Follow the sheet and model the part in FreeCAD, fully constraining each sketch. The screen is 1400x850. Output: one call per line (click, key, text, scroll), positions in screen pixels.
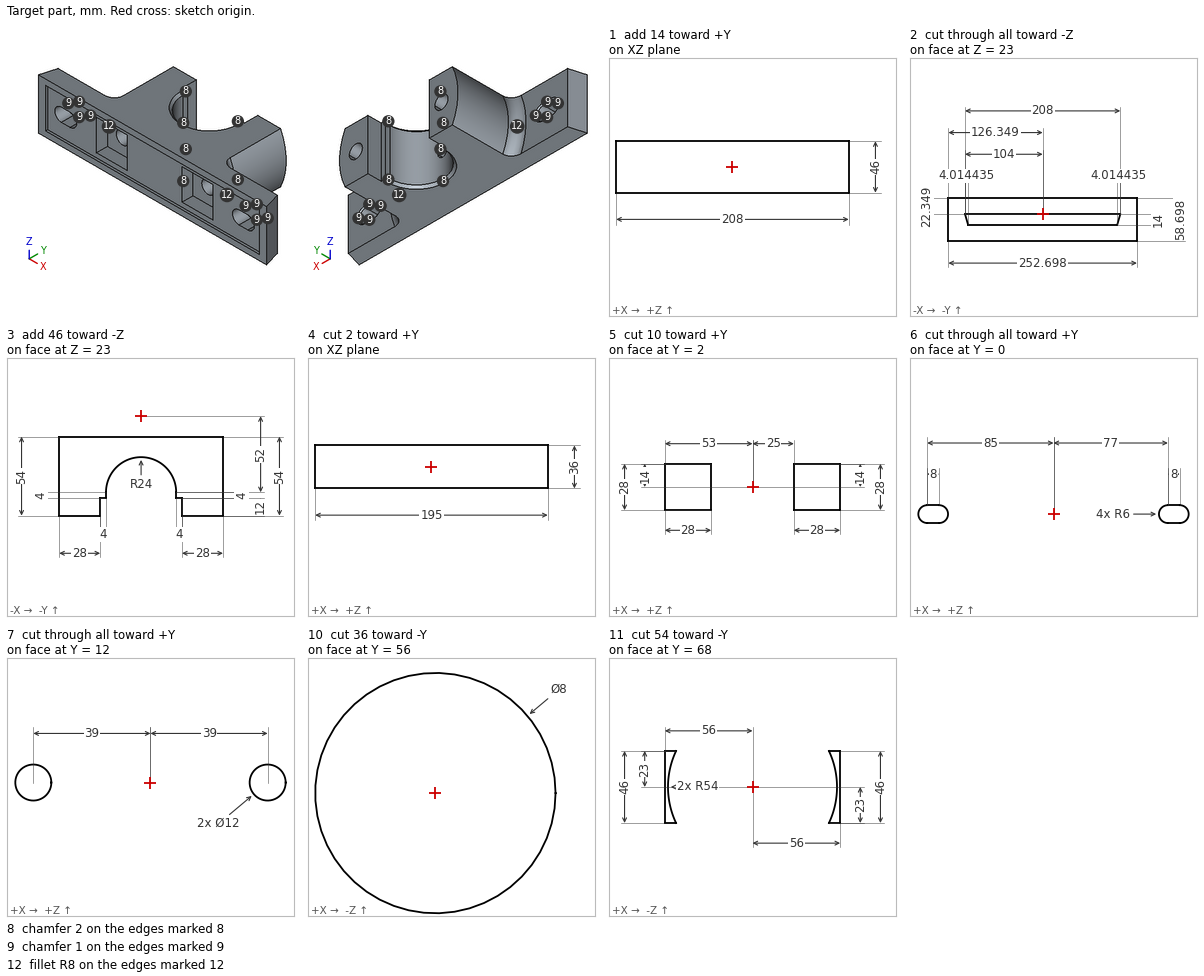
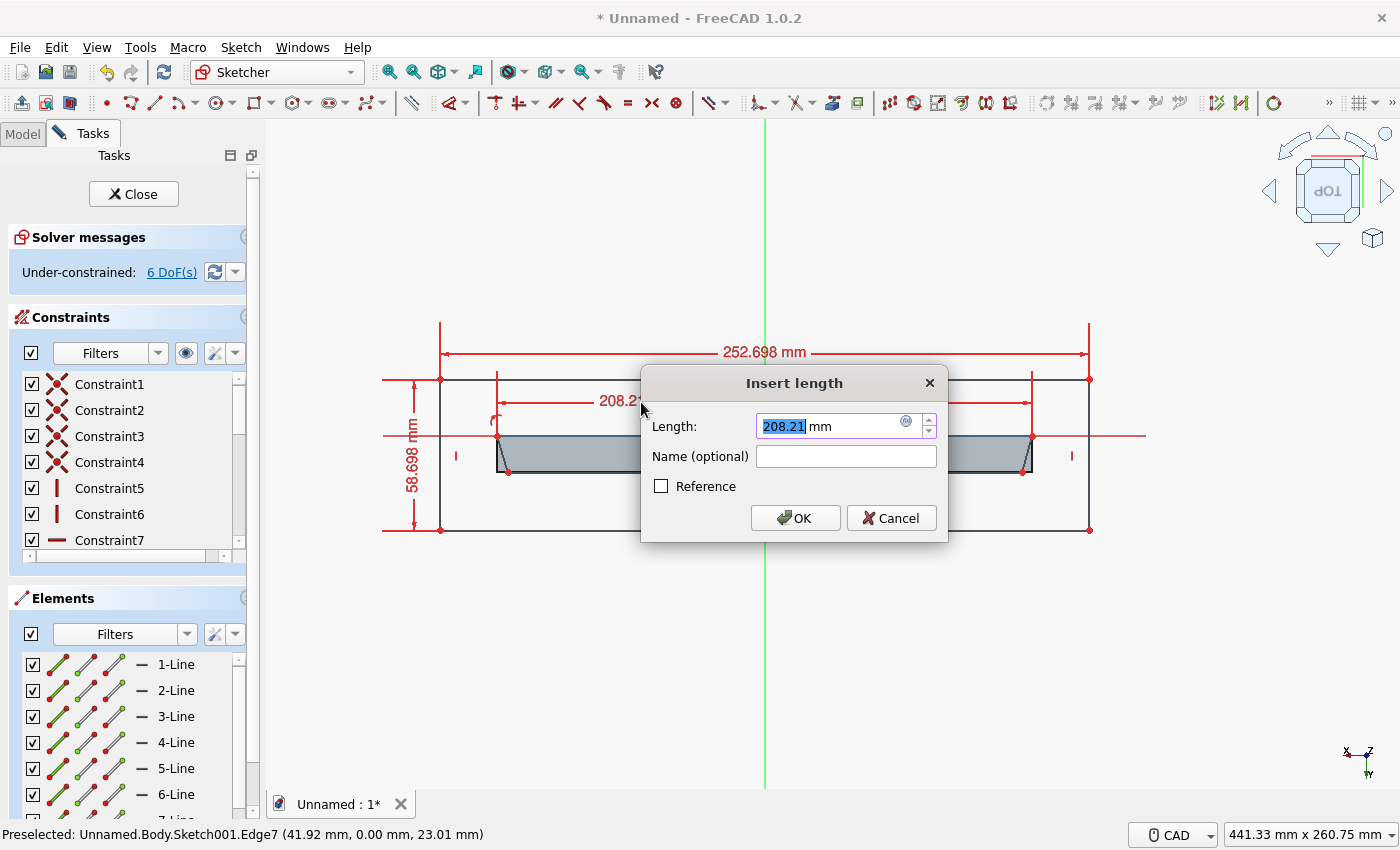
text(208)
key(Return)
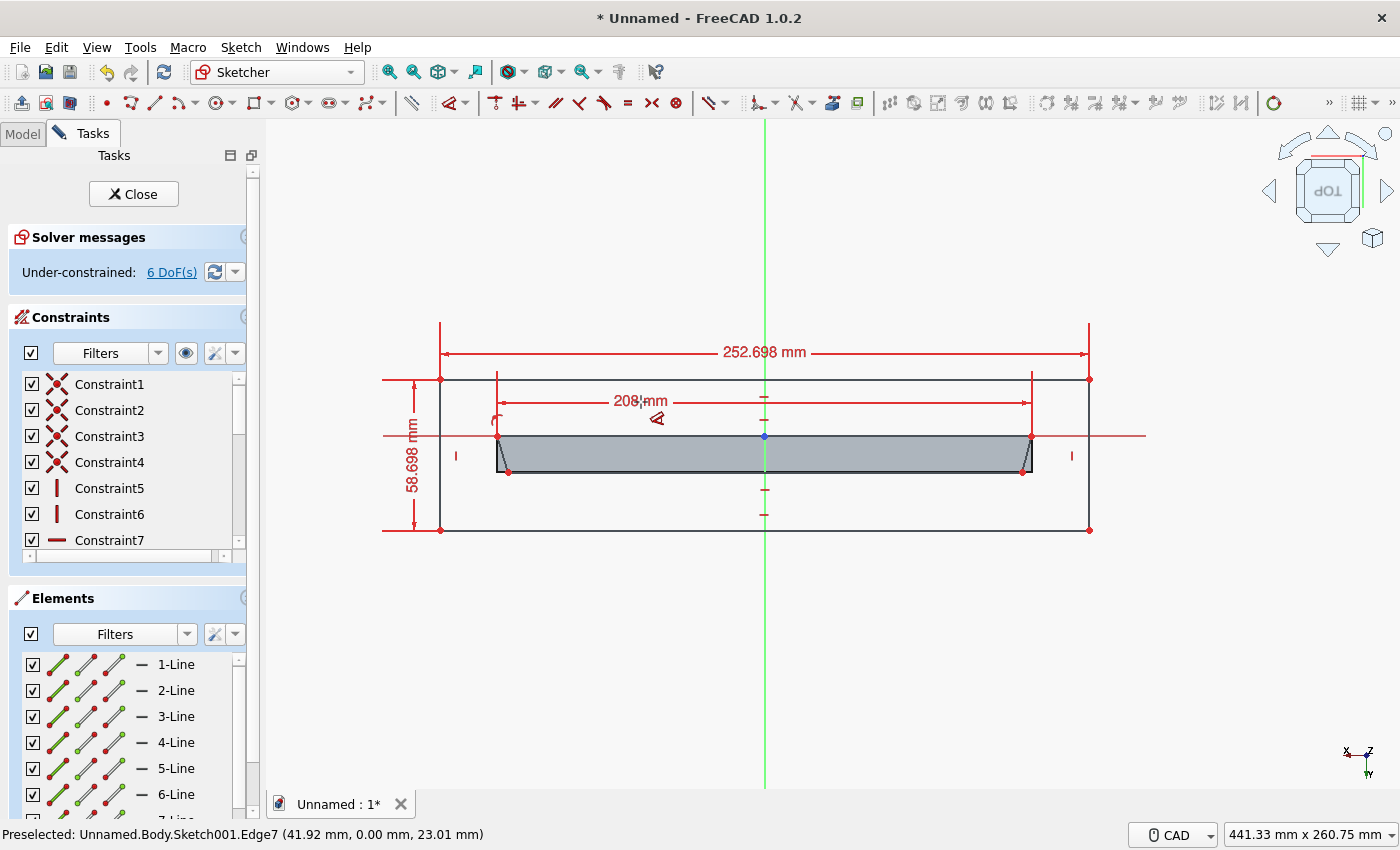
click(1022, 473)
click(1056, 455)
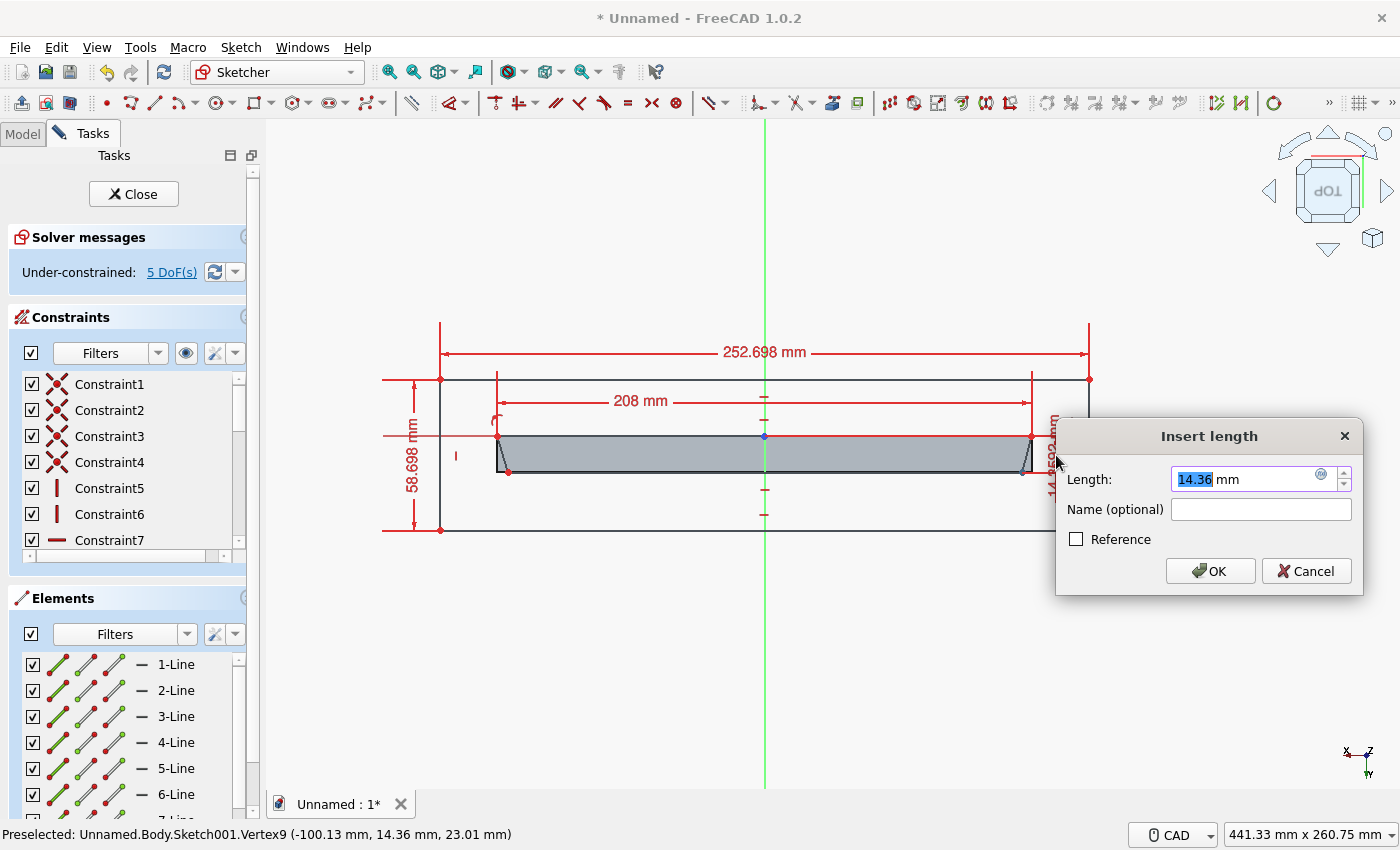
text(14)
key(Return)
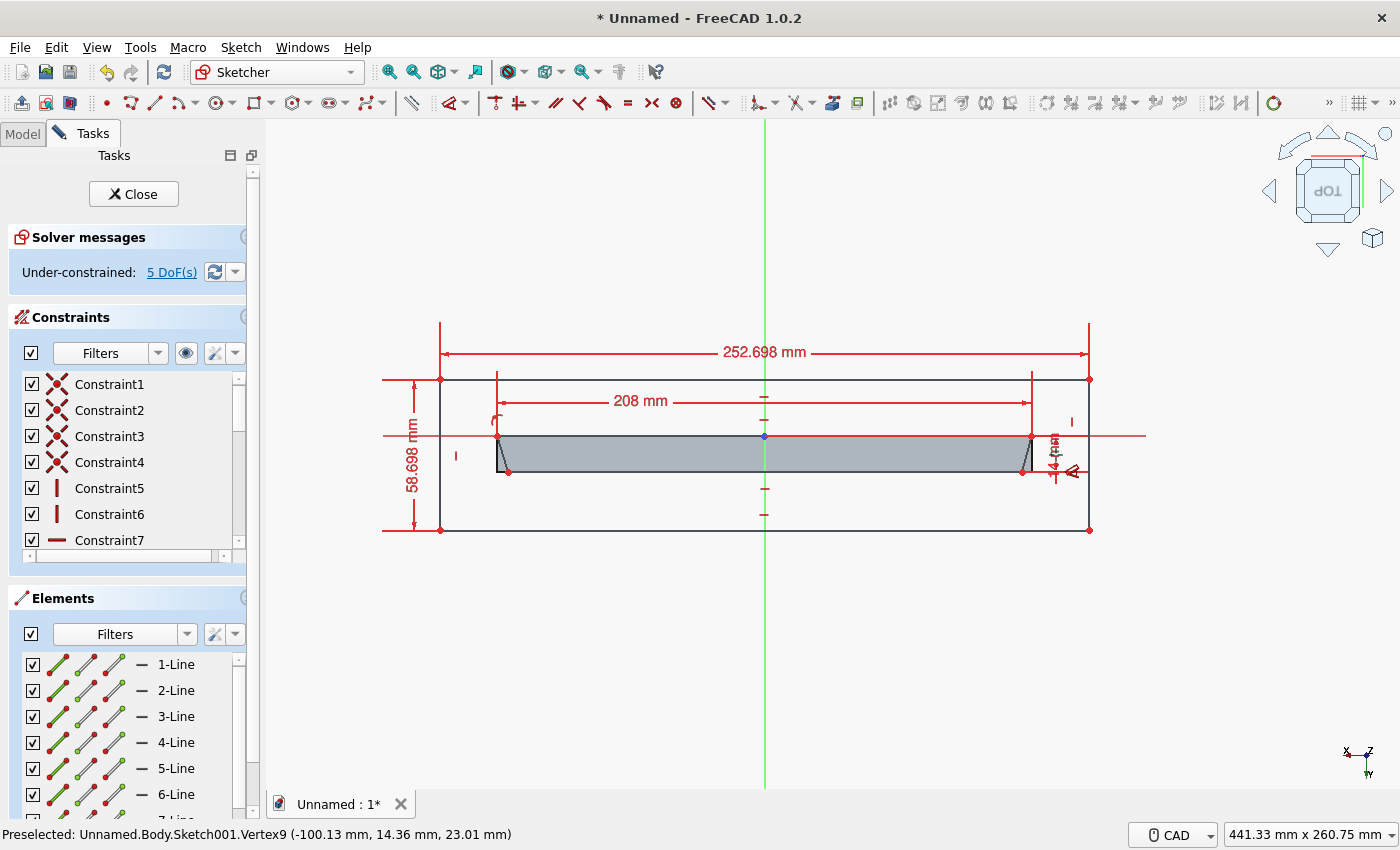
click(497, 436)
click(569, 402)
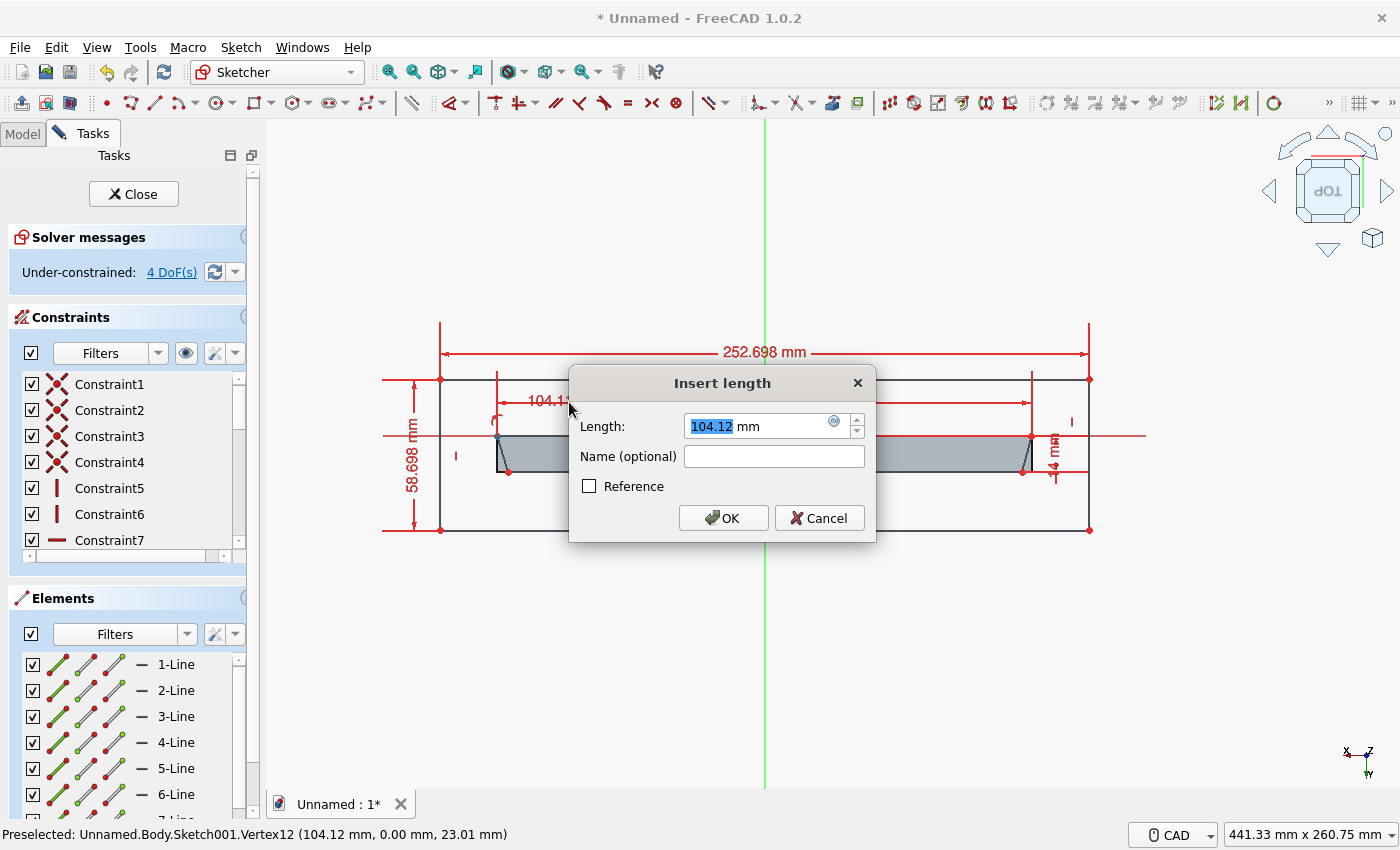
text(104)
key(Return)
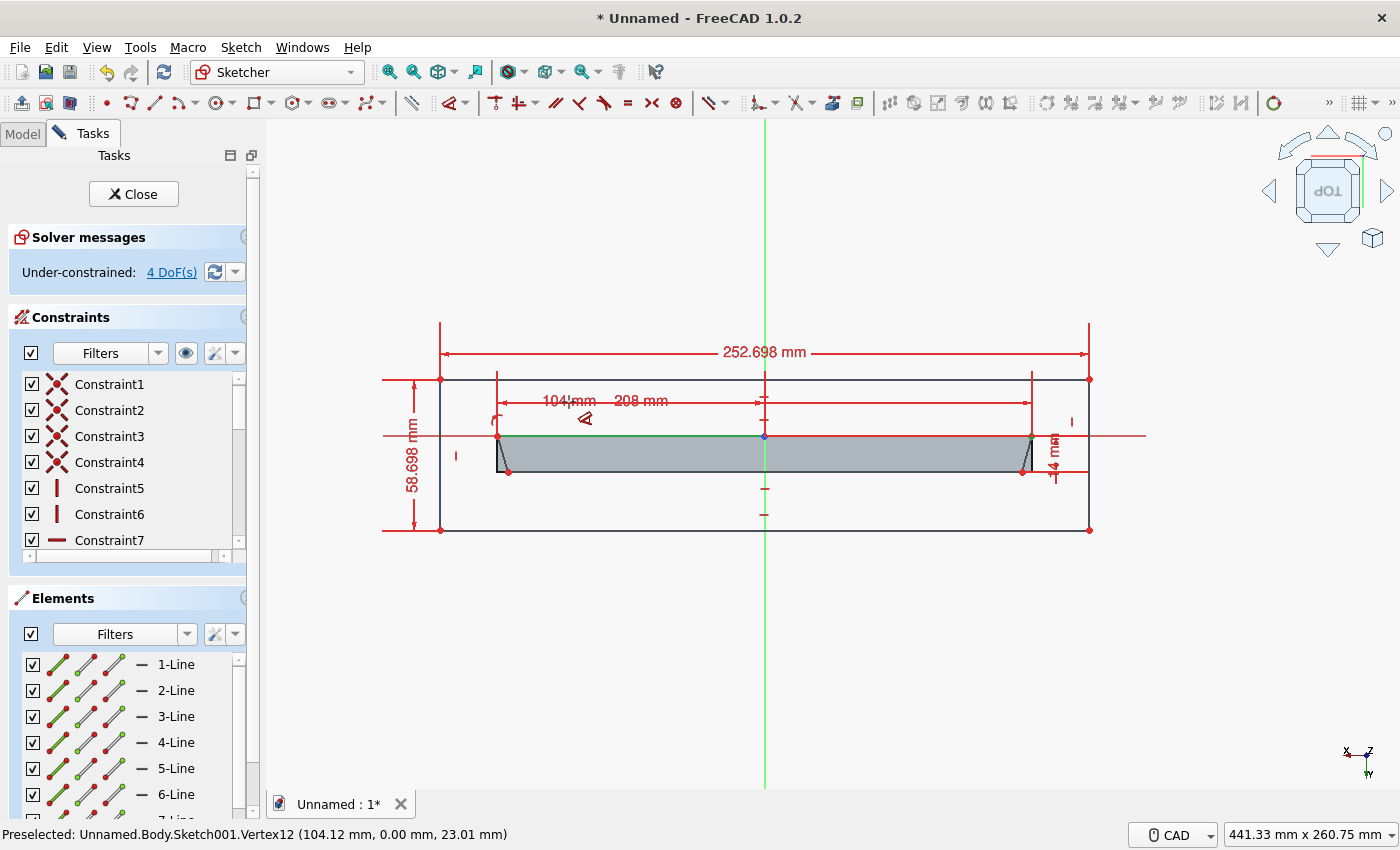
click(440, 380)
click(406, 408)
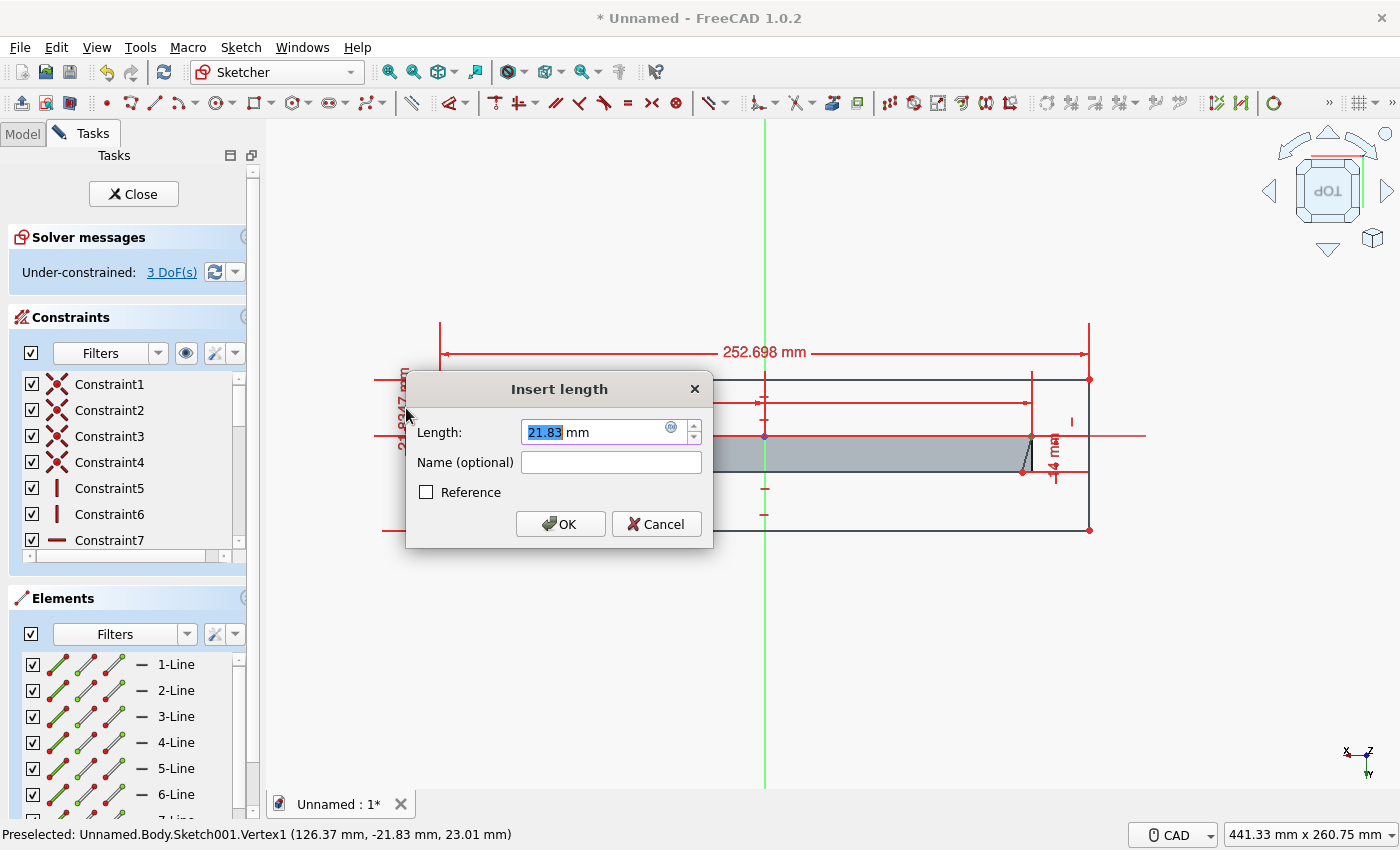
text(22.349)
key(Return)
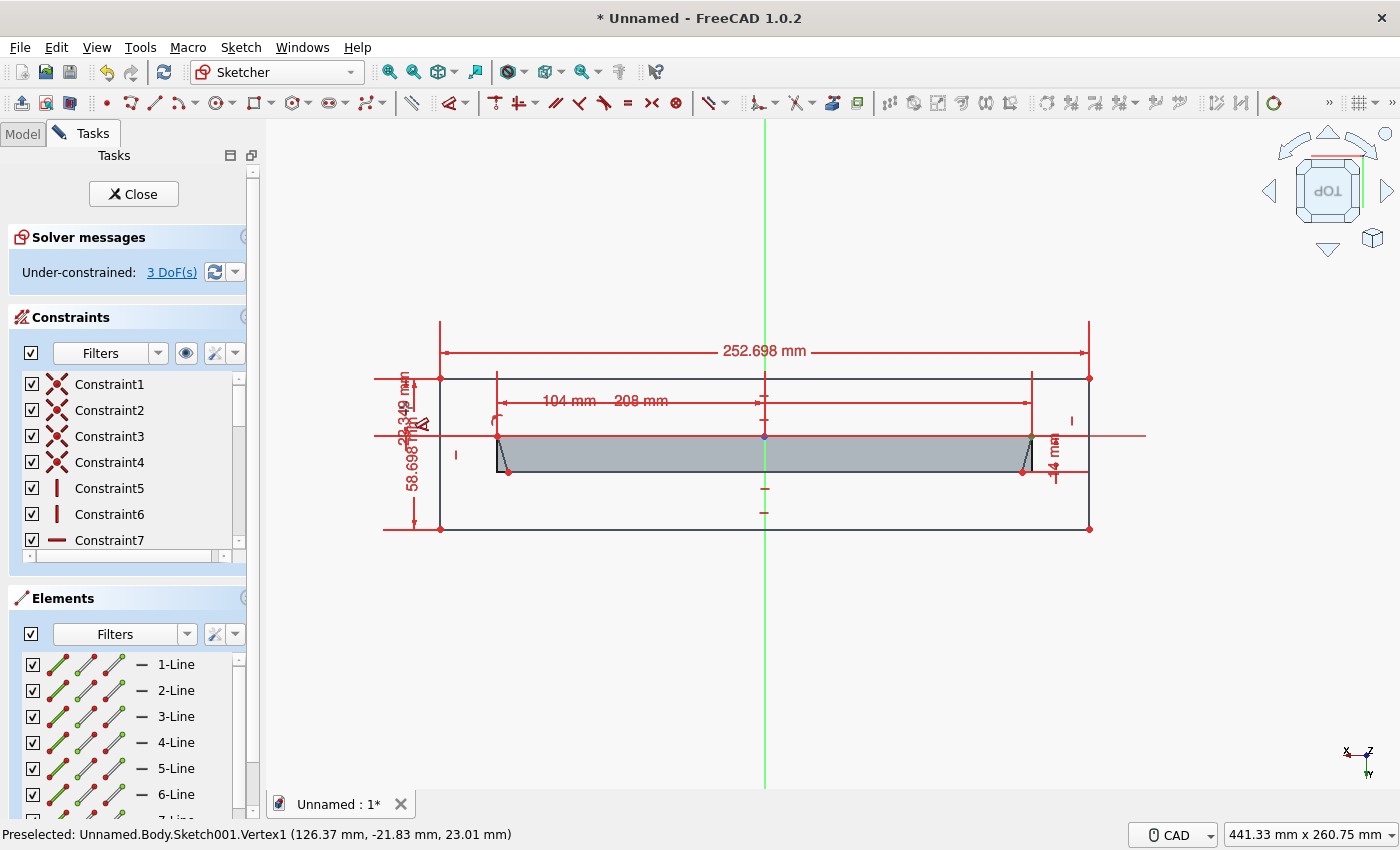
click(440, 379)
click(602, 345)